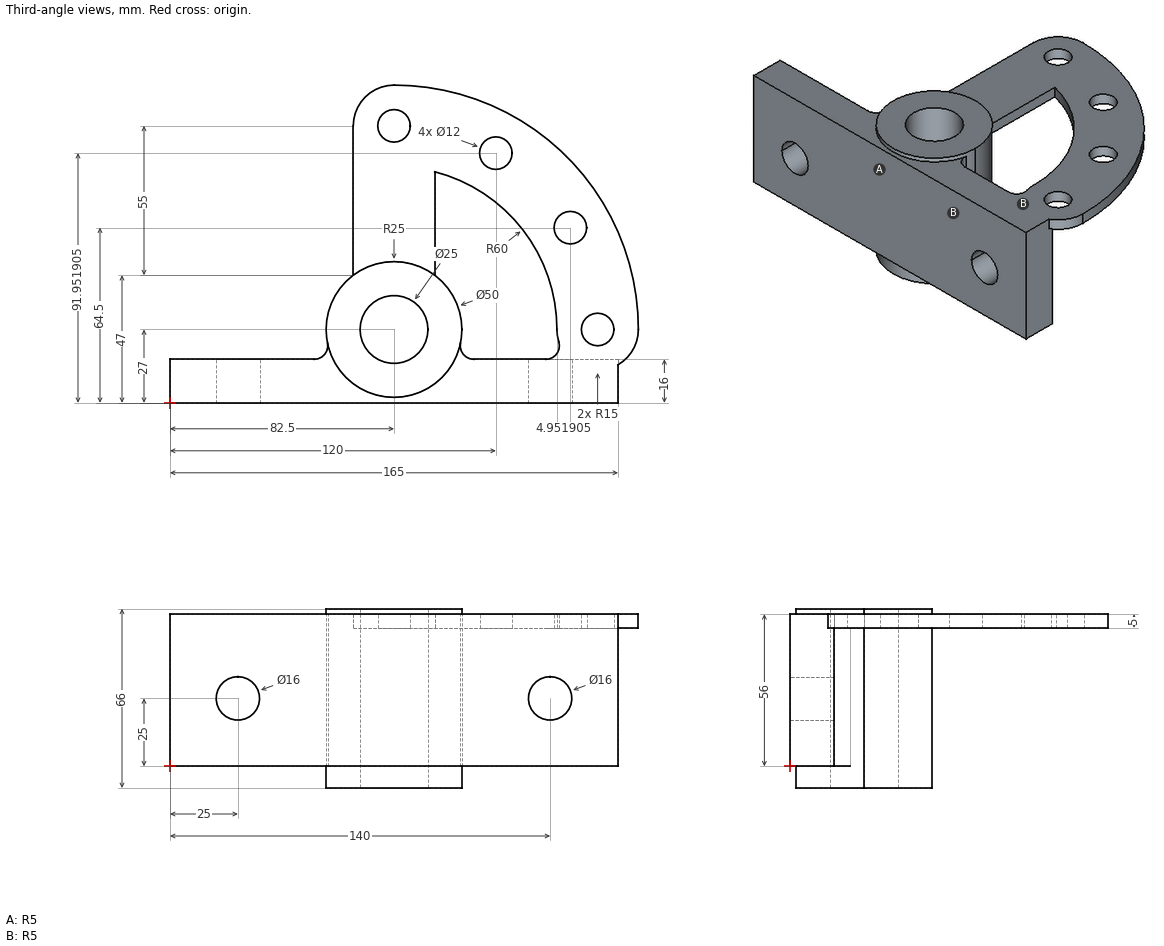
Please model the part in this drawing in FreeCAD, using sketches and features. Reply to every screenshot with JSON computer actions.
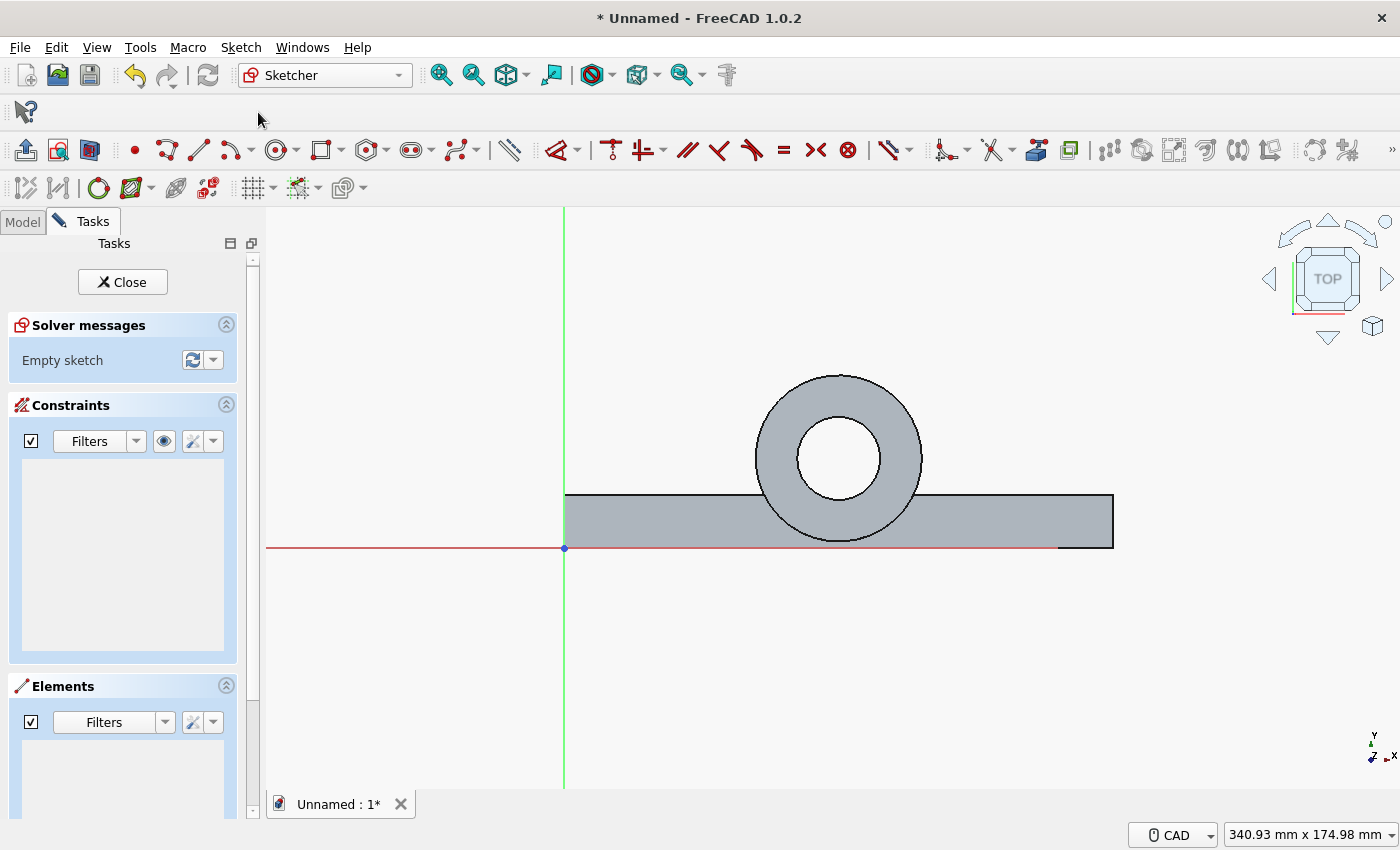
{"action": "left_click", "coordinate": [90, 150]}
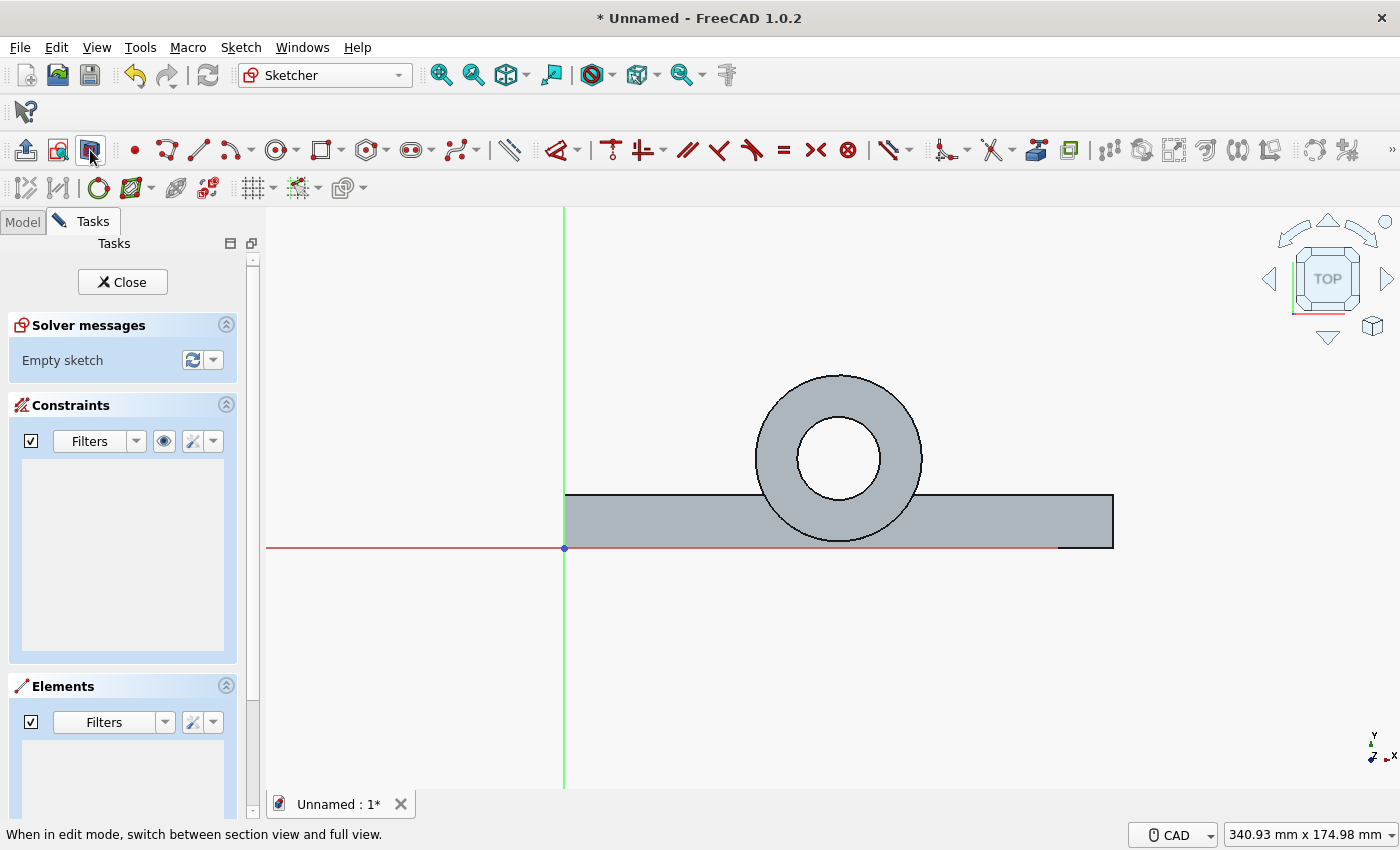
{"action": "scroll", "coordinate": [373, 761], "scroll_direction": "down", "scroll_amount": 1}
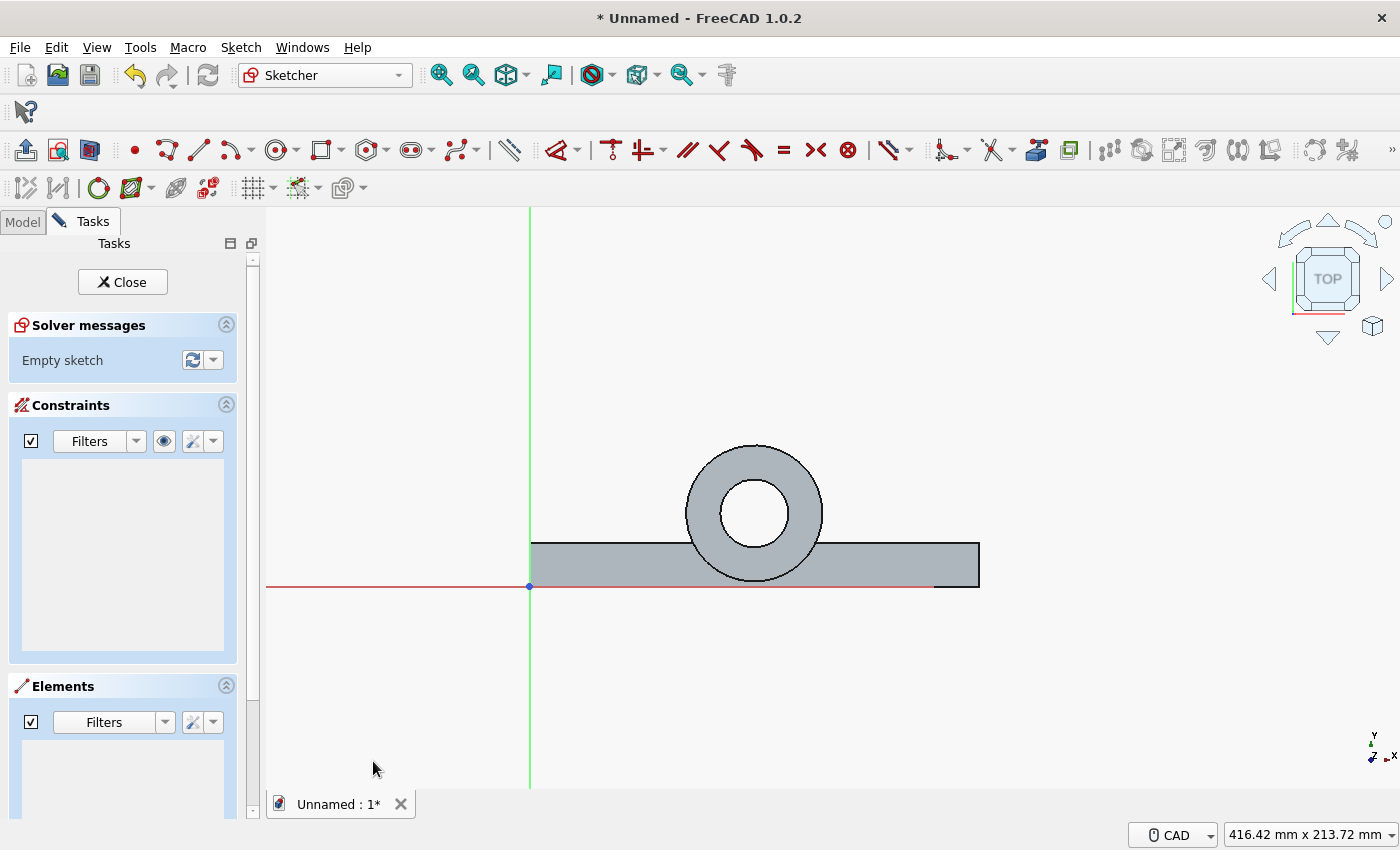
{"action": "left_click", "coordinate": [200, 150]}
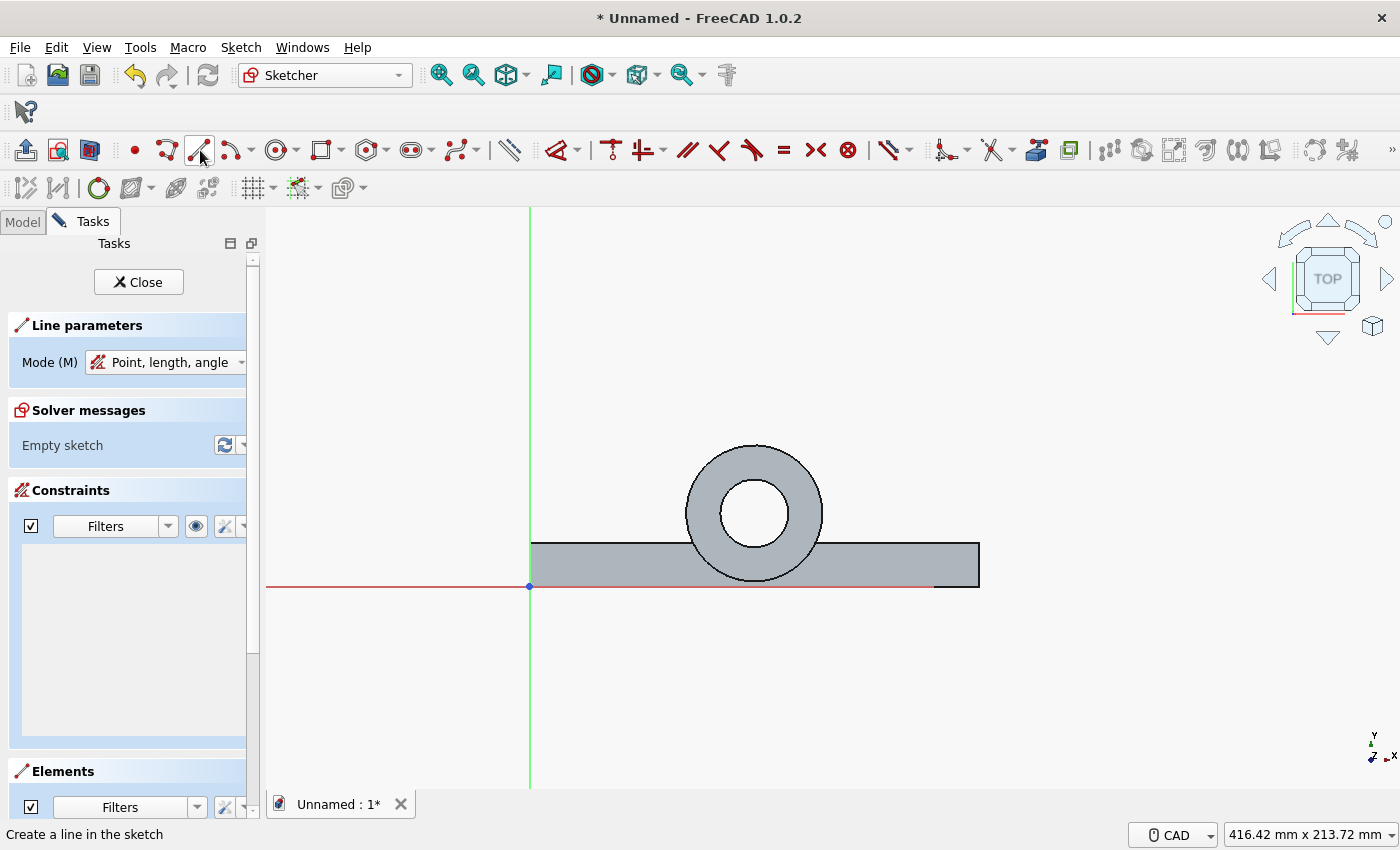
{"action": "left_click", "coordinate": [713, 309]}
{"action": "left_click", "coordinate": [713, 459]}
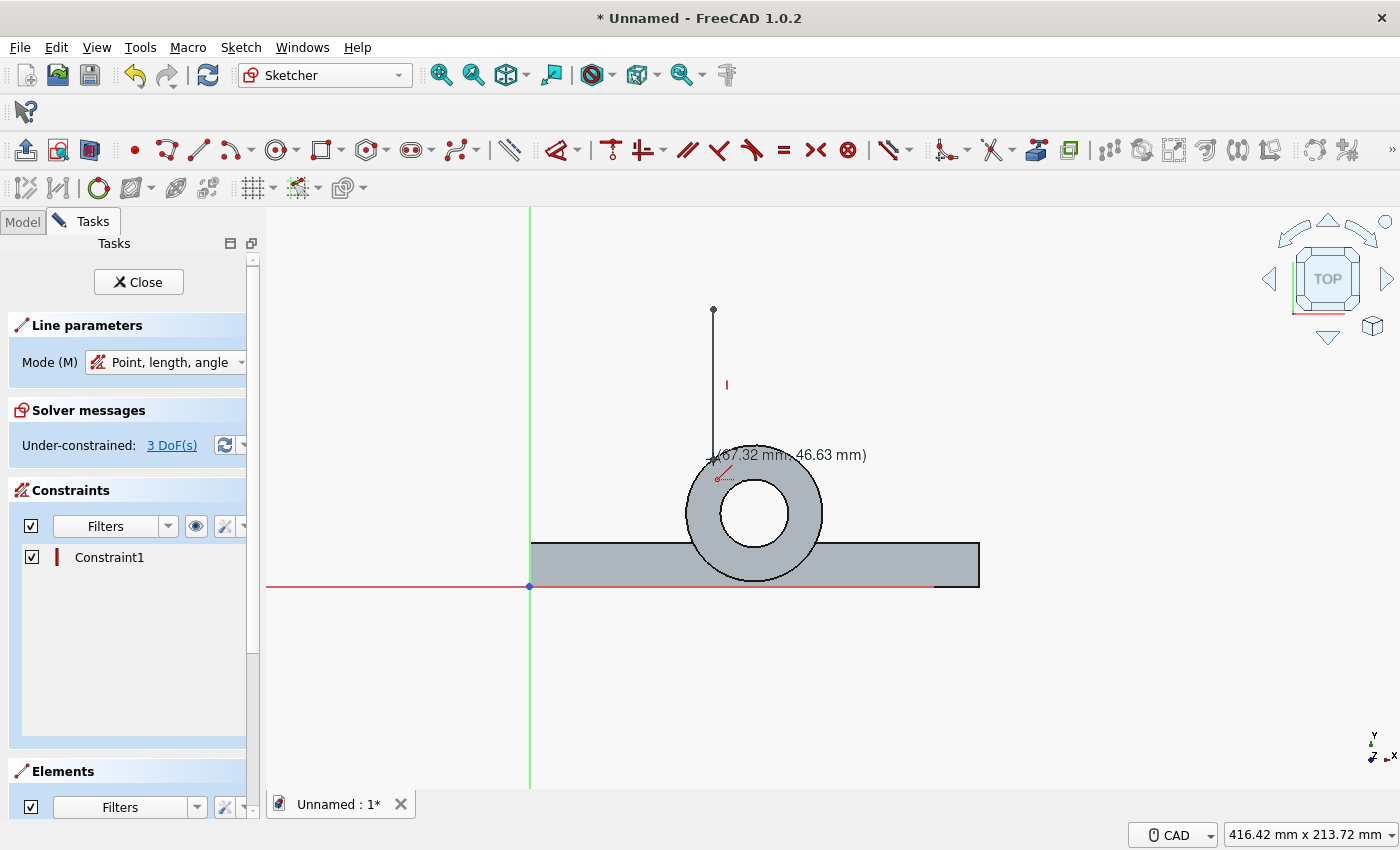
{"action": "left_click", "coordinate": [795, 459]}
{"action": "left_click", "coordinate": [795, 355]}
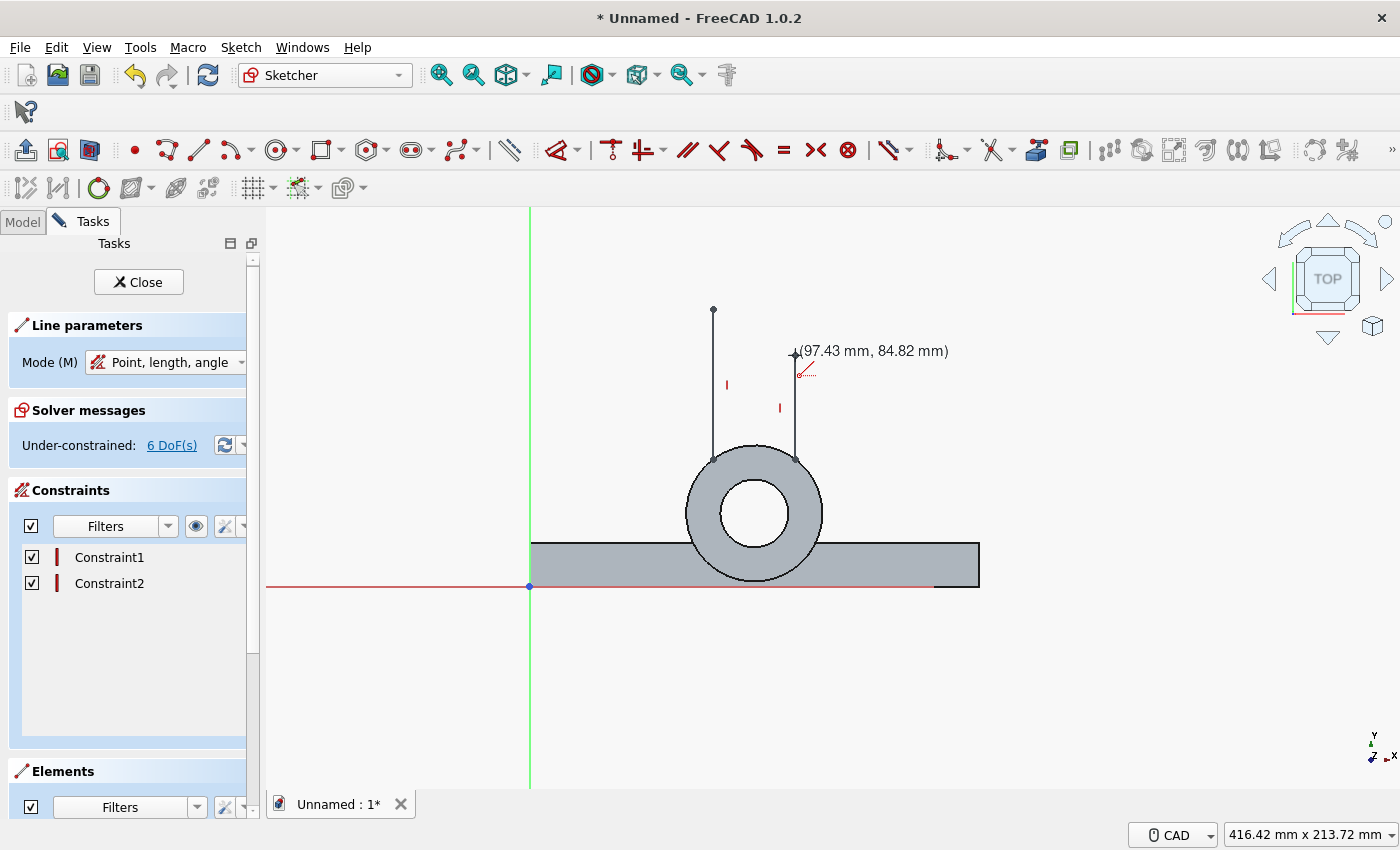
{"action": "left_click", "coordinate": [254, 150]}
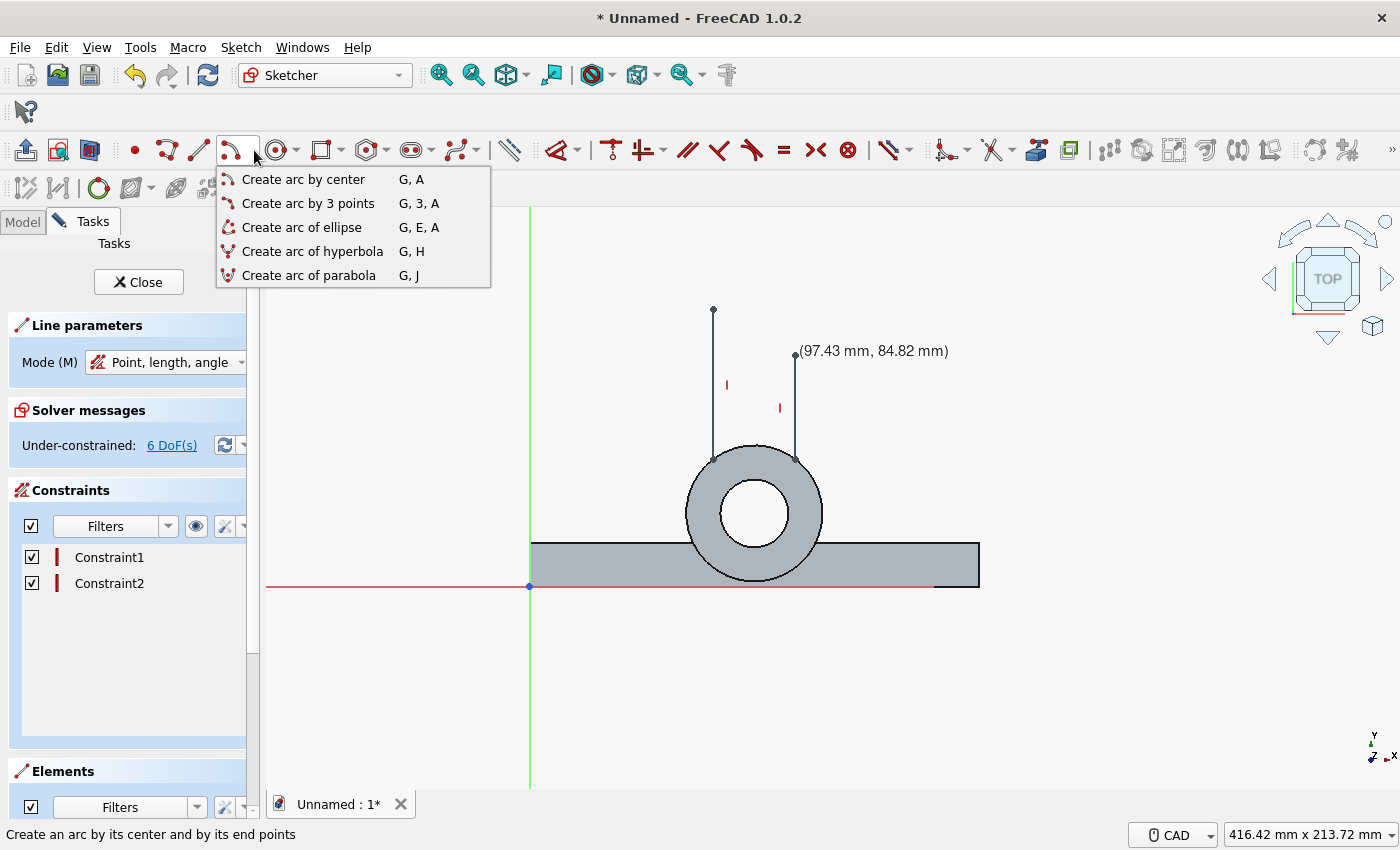
{"action": "left_click", "coordinate": [354, 203]}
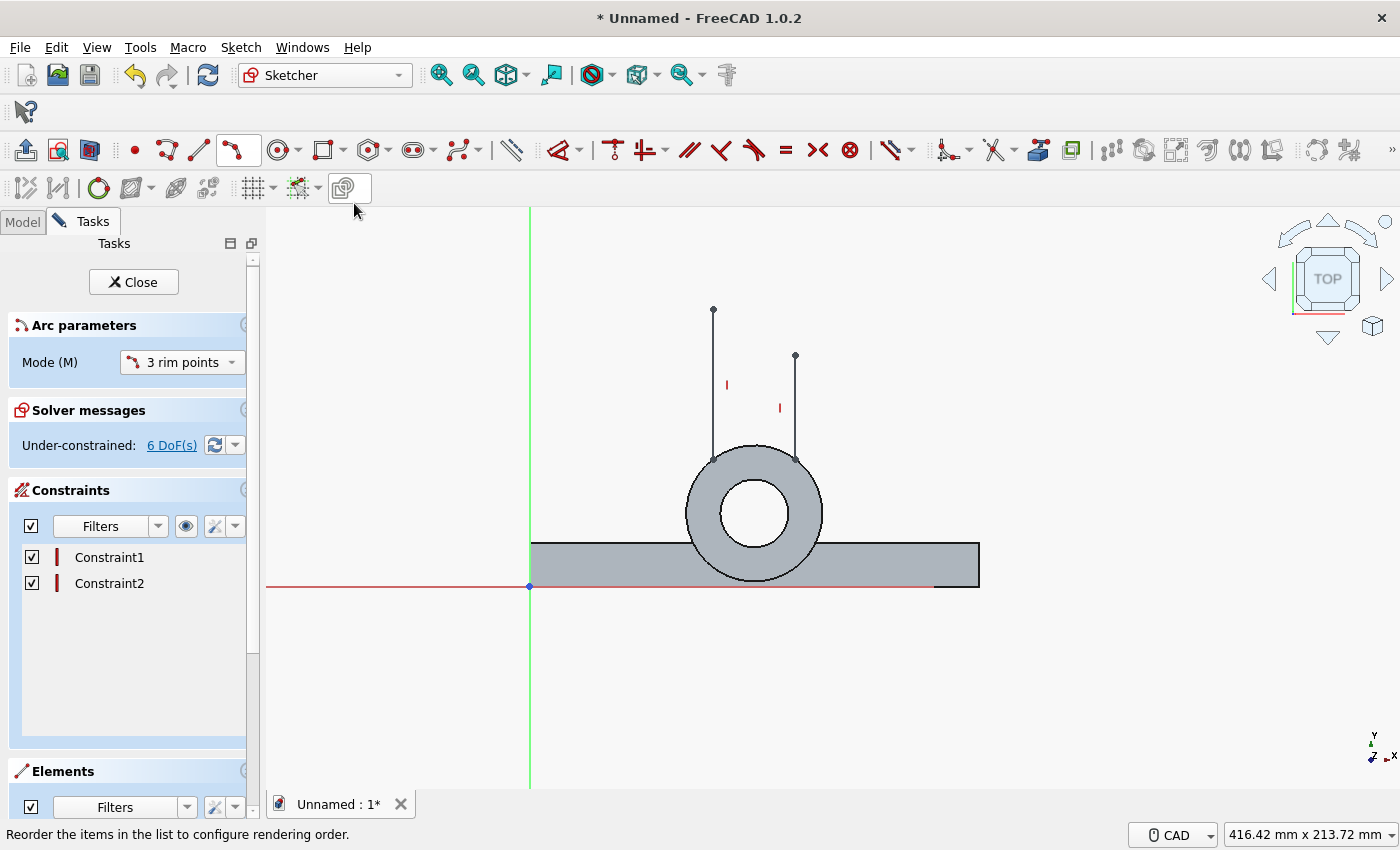
{"action": "left_click", "coordinate": [713, 460]}
{"action": "left_click", "coordinate": [795, 460]}
{"action": "left_click", "coordinate": [754, 445]}